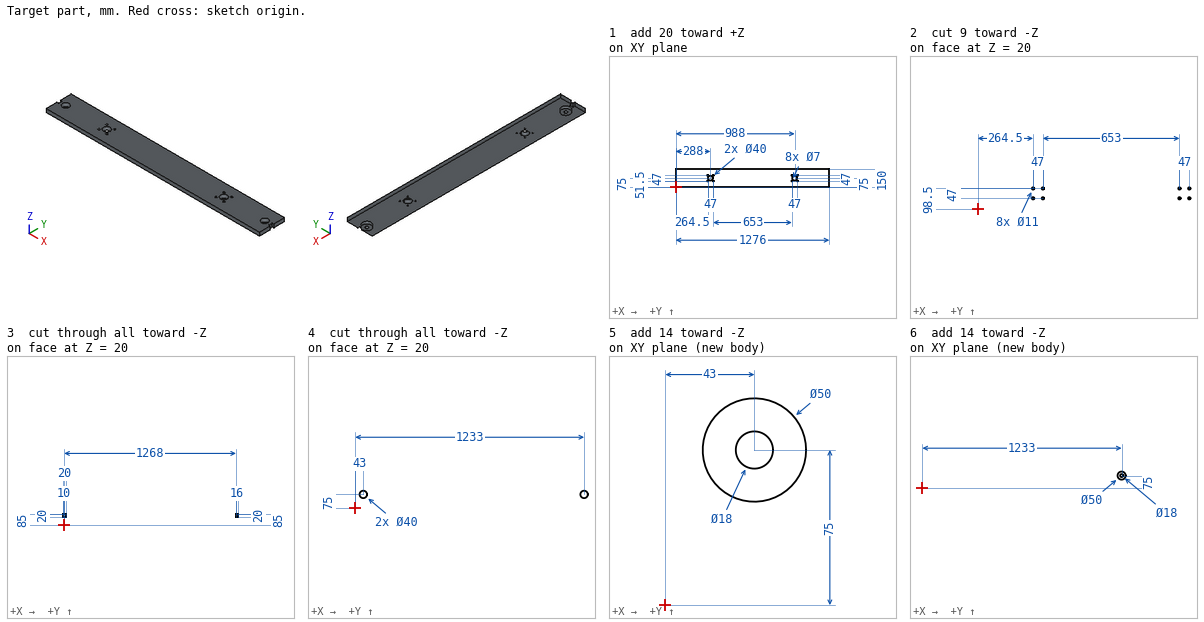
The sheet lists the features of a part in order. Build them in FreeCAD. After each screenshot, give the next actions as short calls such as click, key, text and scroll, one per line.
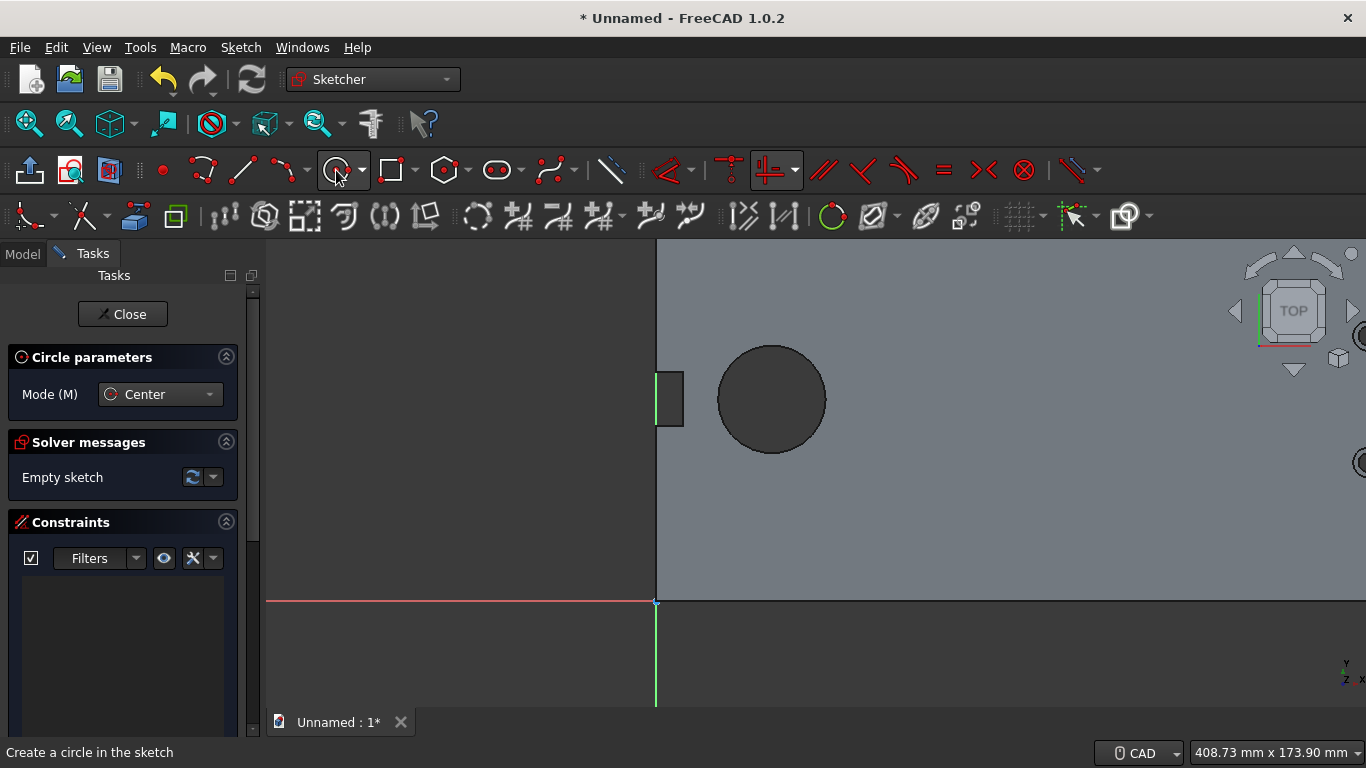
click(772, 399)
move(819, 352)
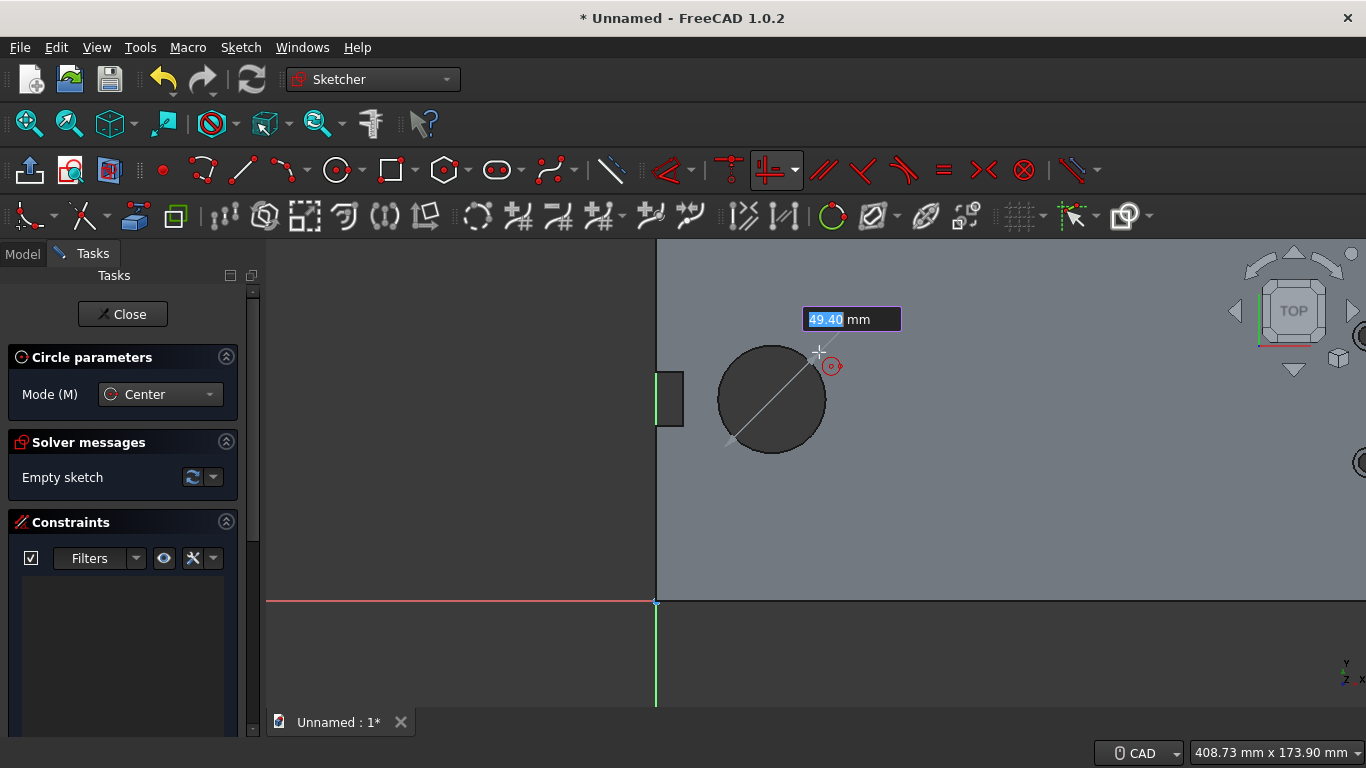
text(50)
key(Return)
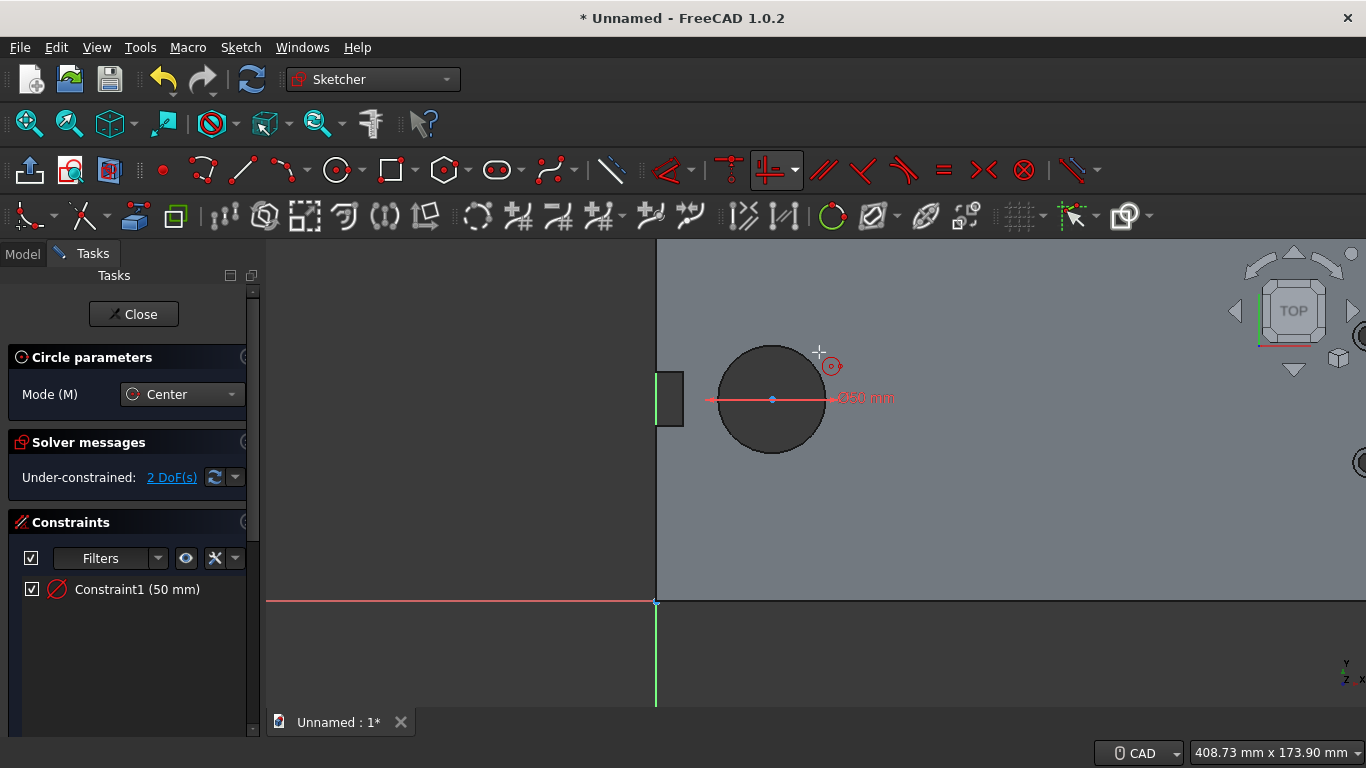
click(772, 400)
move(789, 382)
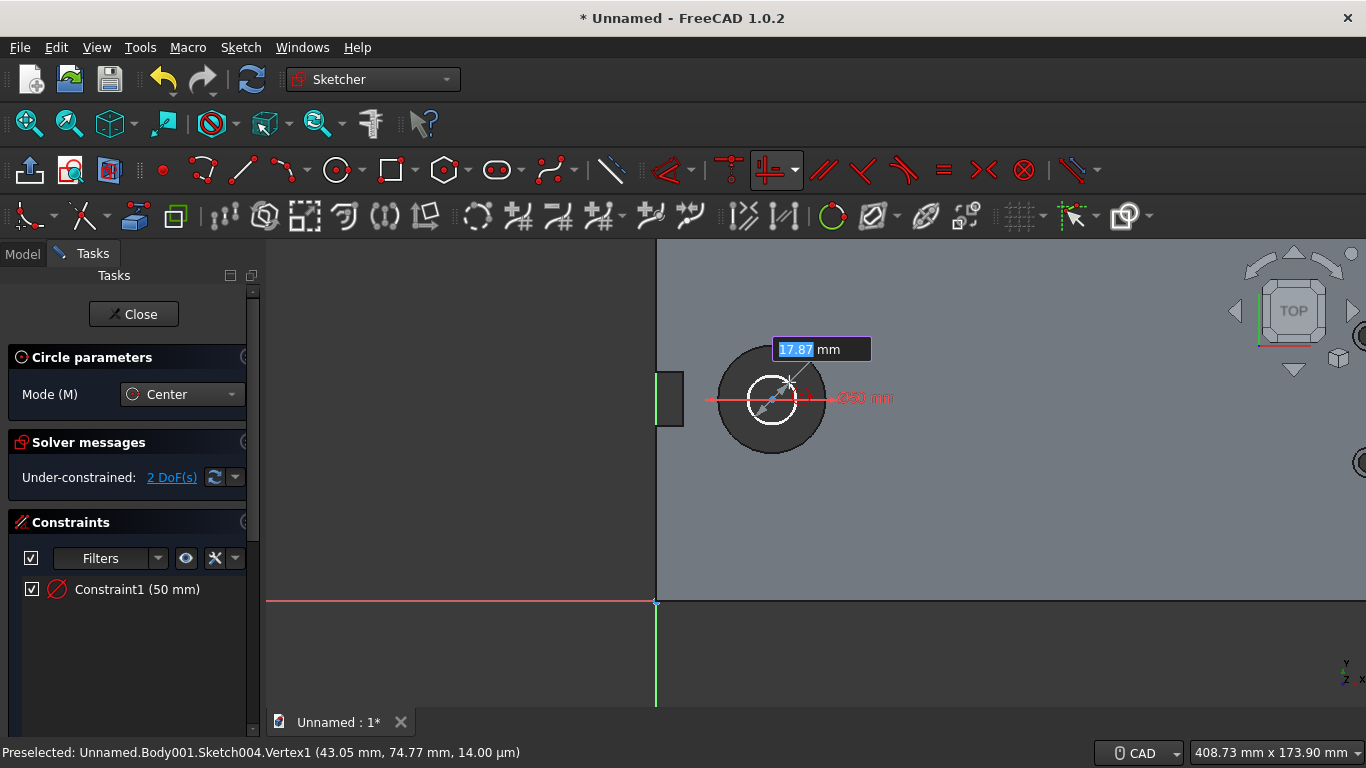
text(18)
key(Return)
key(Escape)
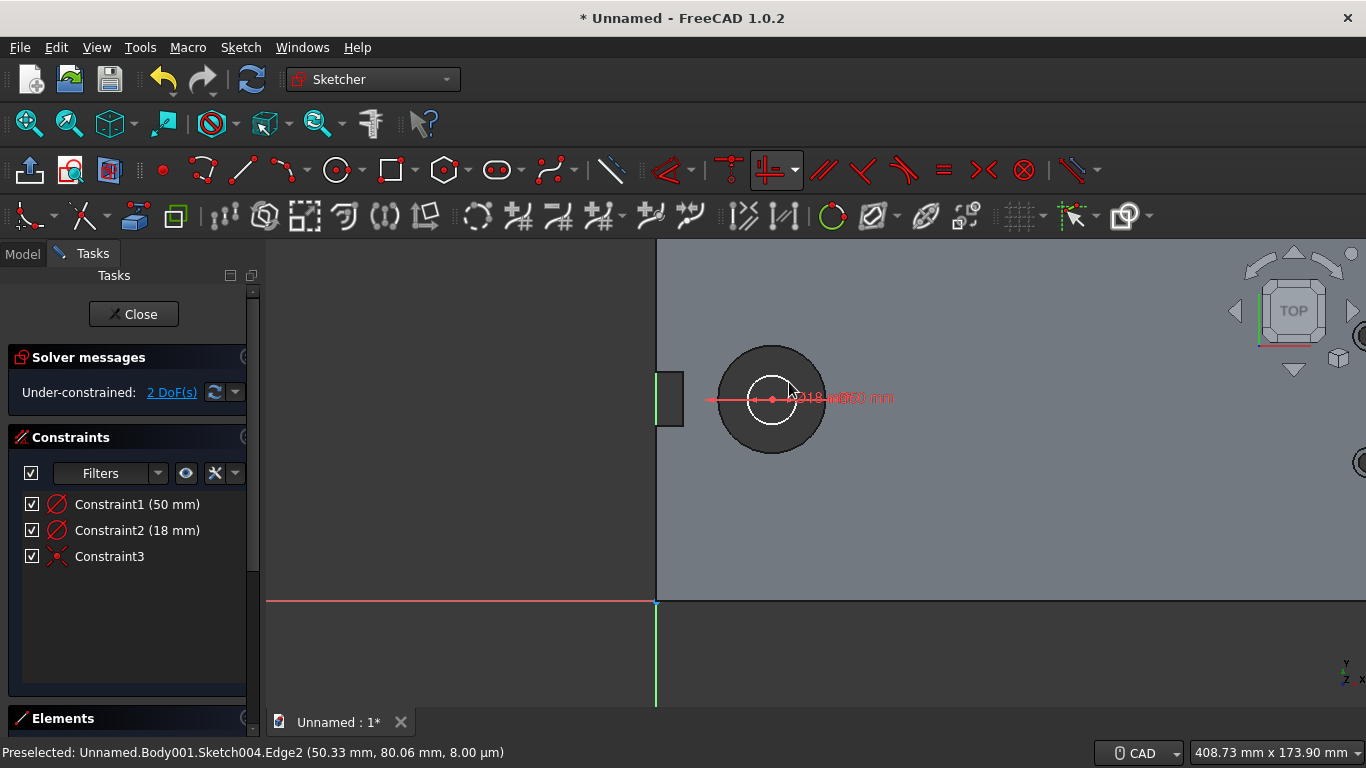
click(666, 170)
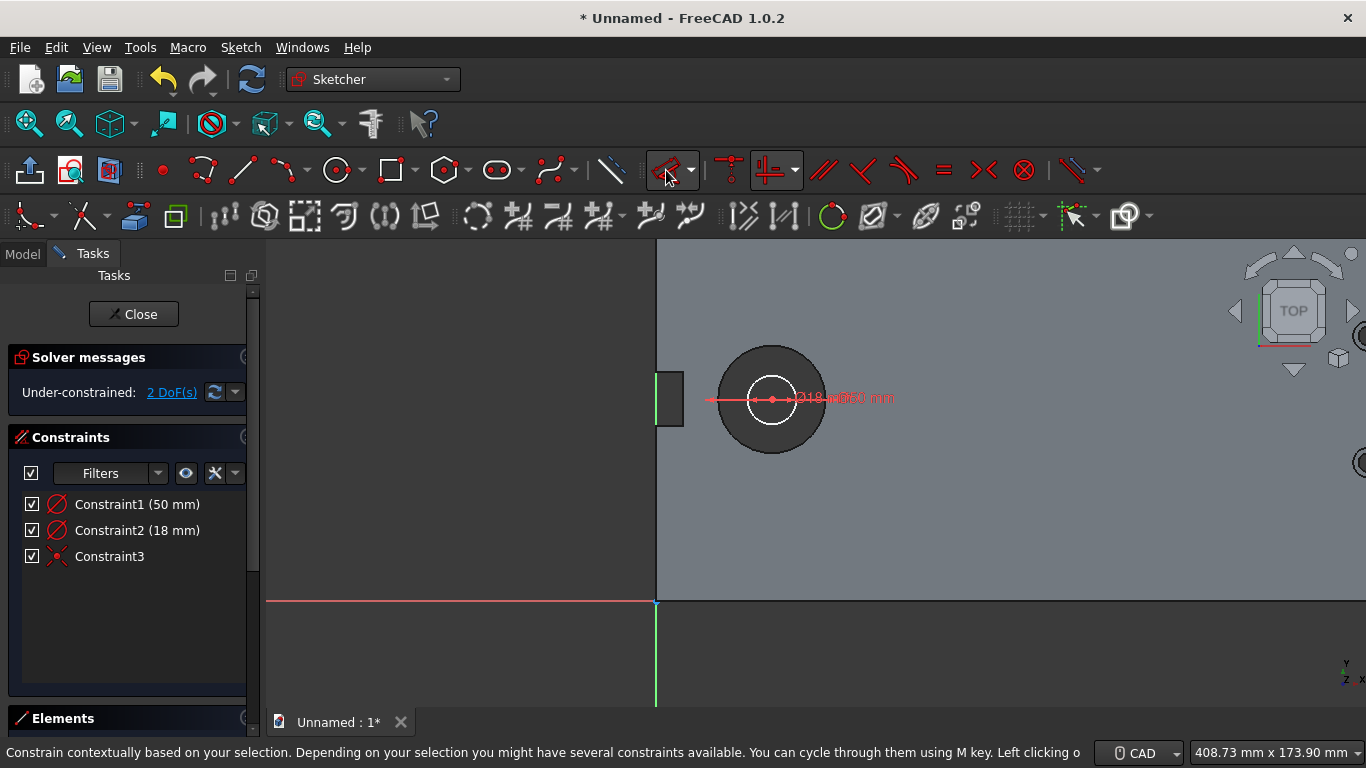
click(772, 400)
click(714, 635)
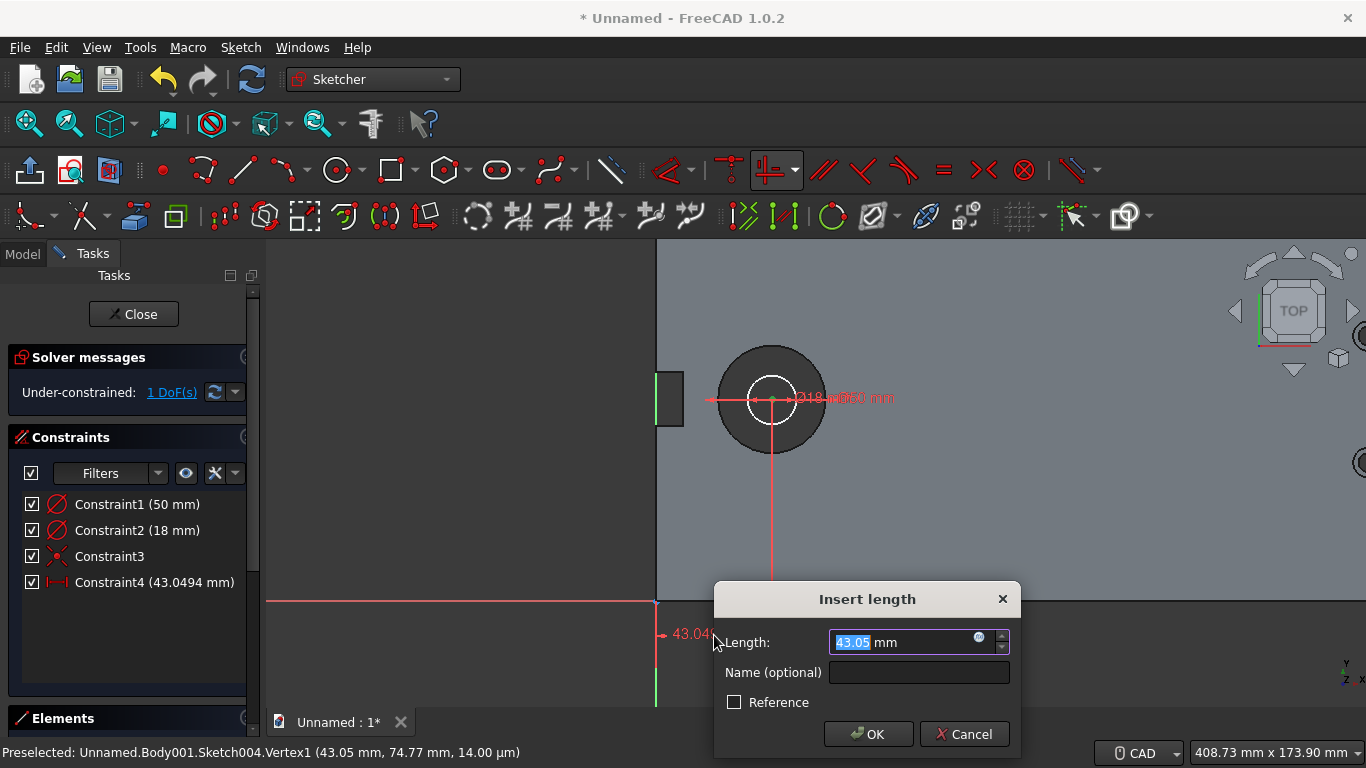
text(43)
key(Return)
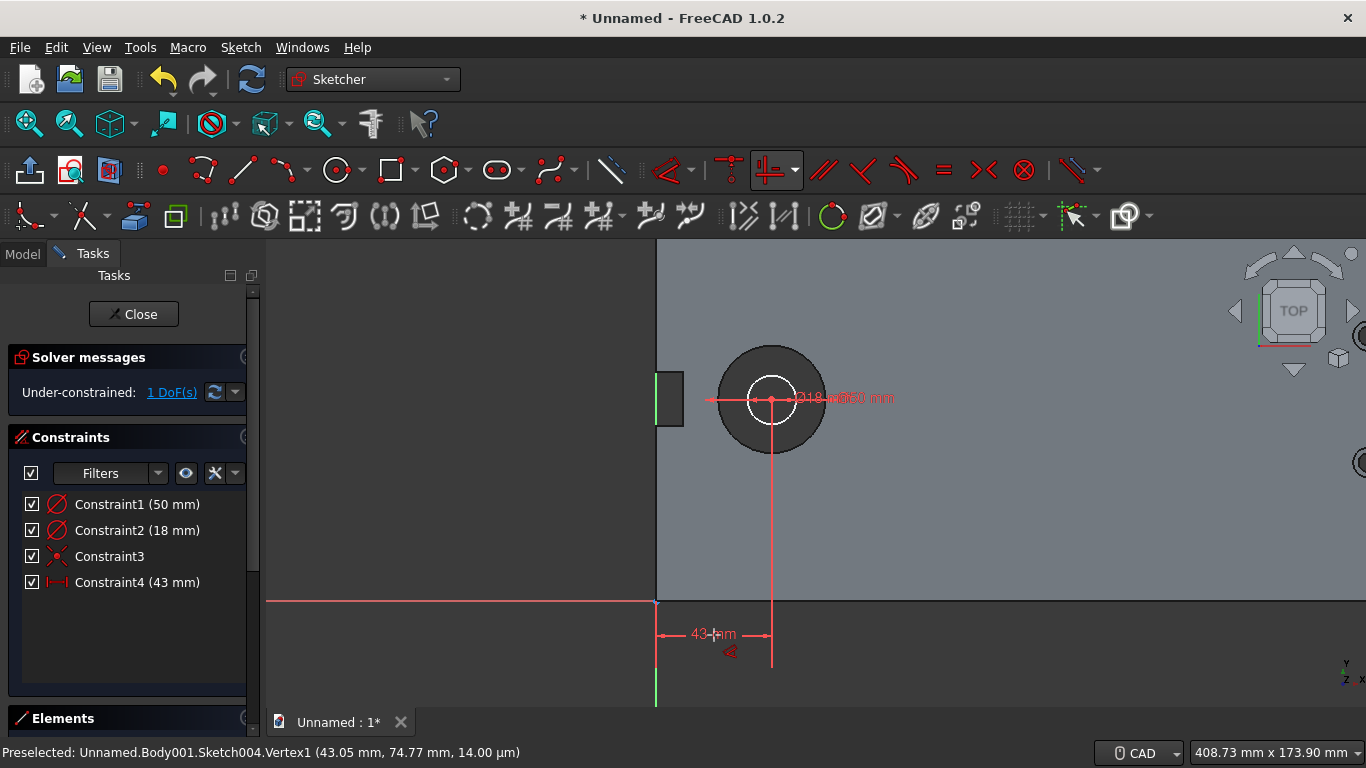
click(772, 400)
click(622, 501)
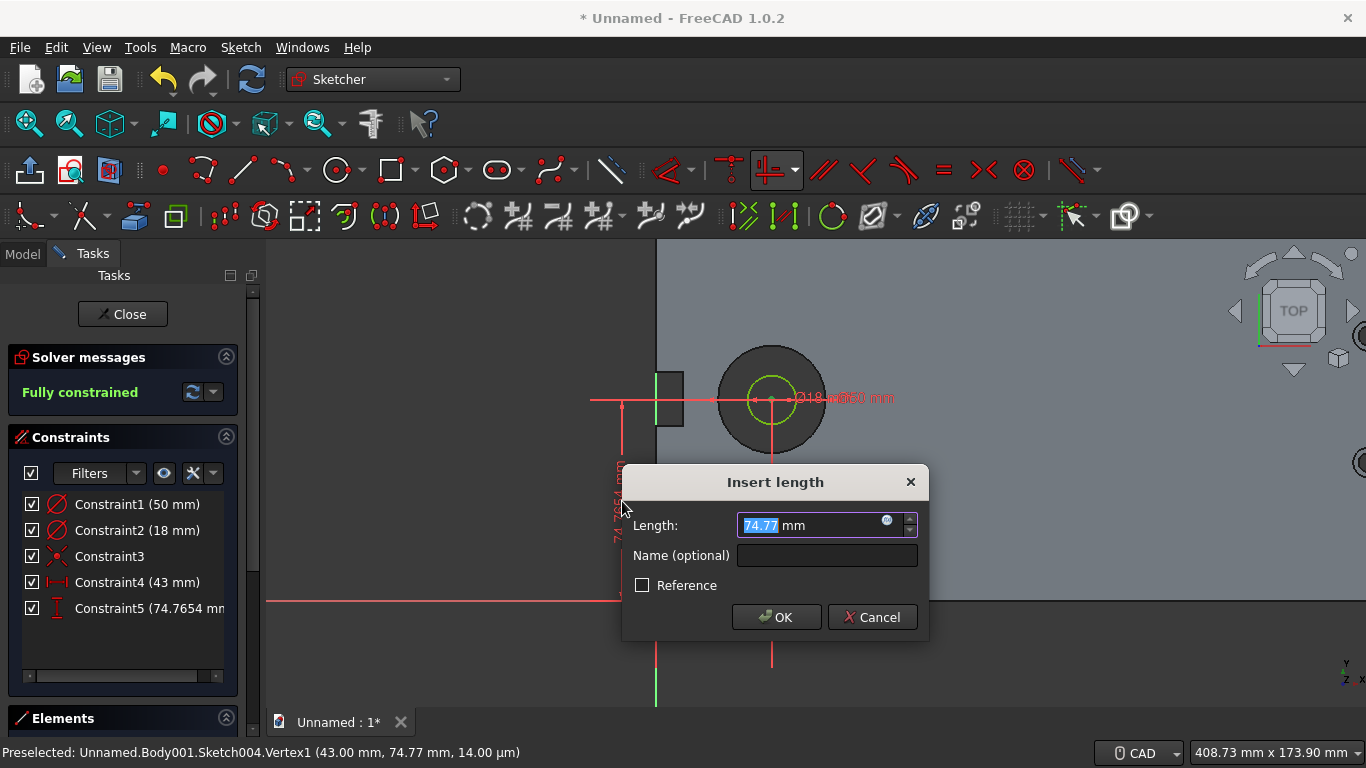
text(75)
key(Return)
key(Escape)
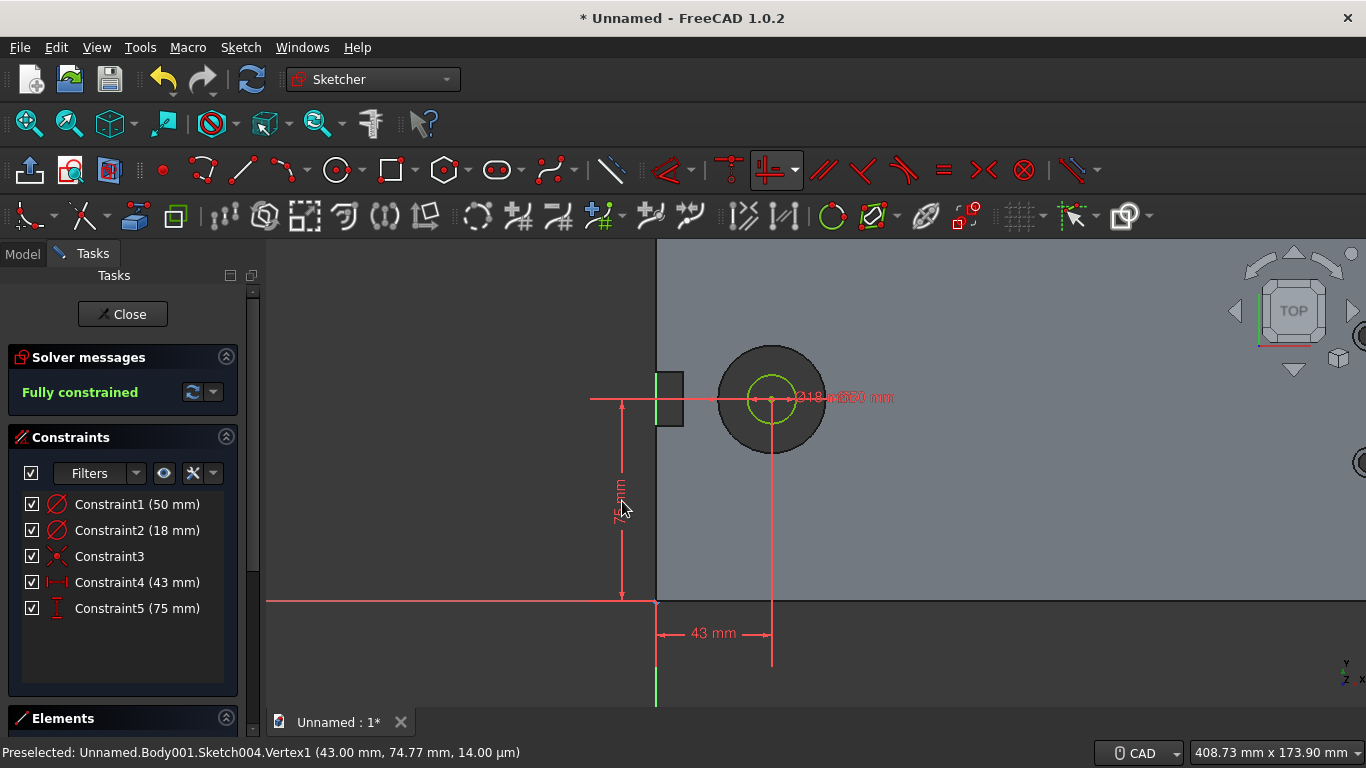
click(123, 314)